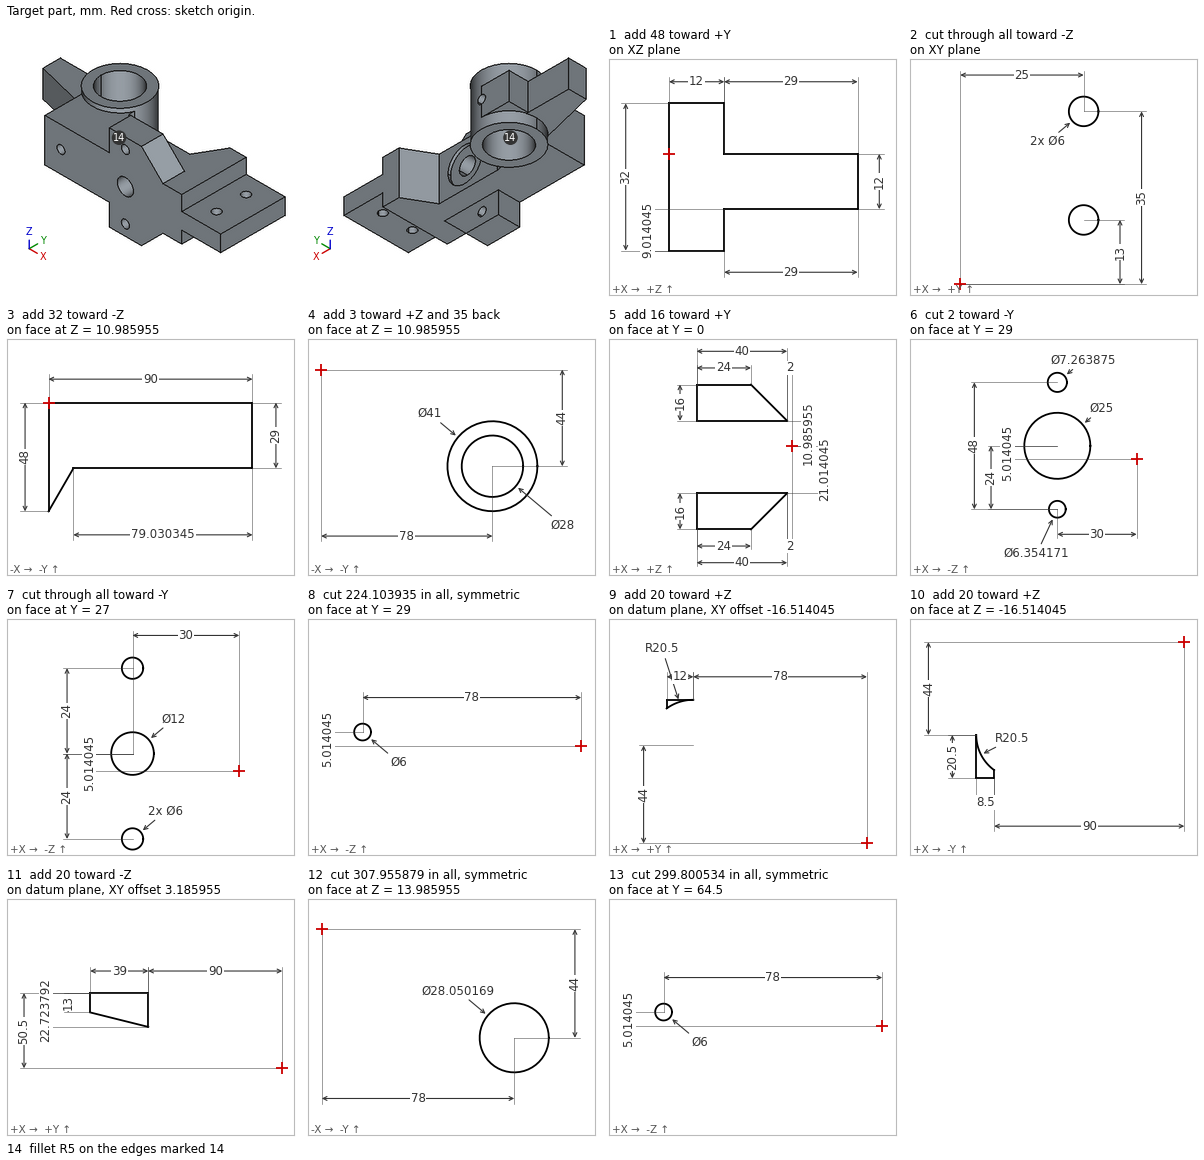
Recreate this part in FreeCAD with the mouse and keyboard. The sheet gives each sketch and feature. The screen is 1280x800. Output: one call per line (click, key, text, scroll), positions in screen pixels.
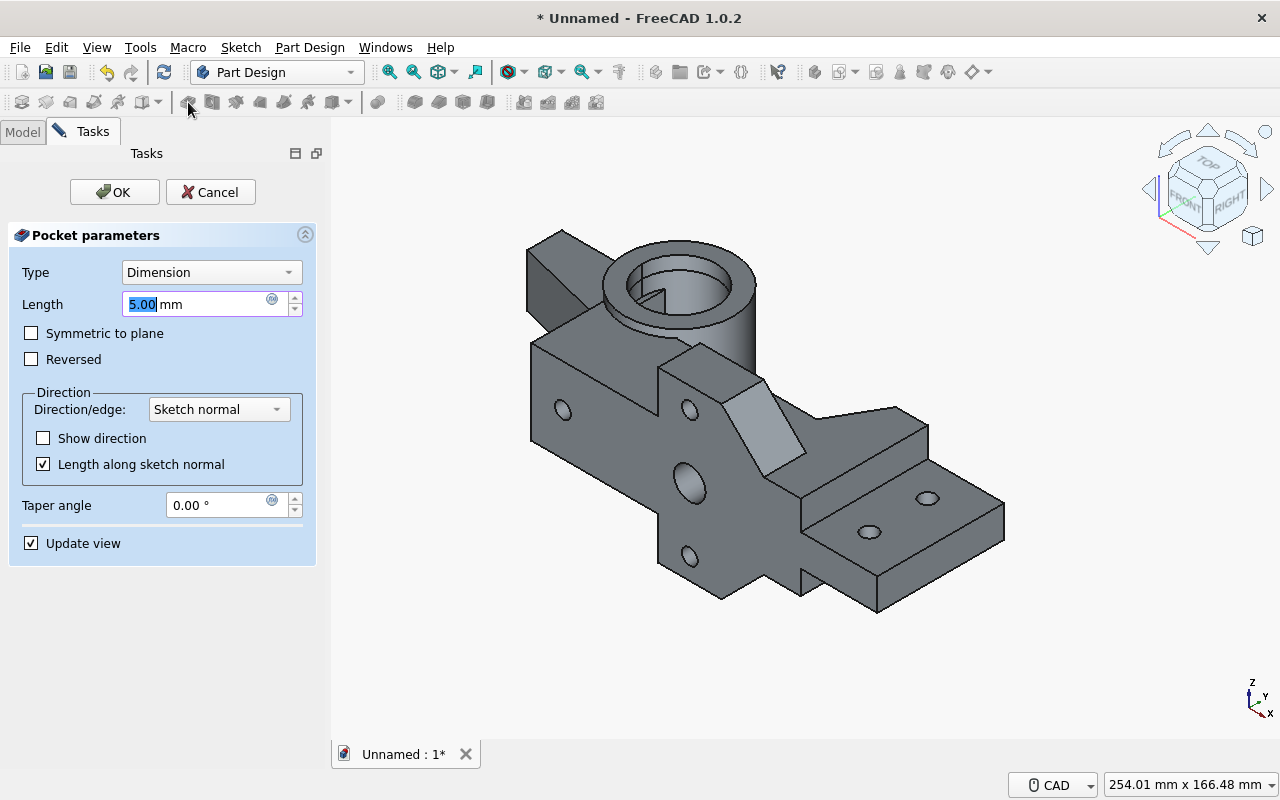
text(307.955879)
key(Tab)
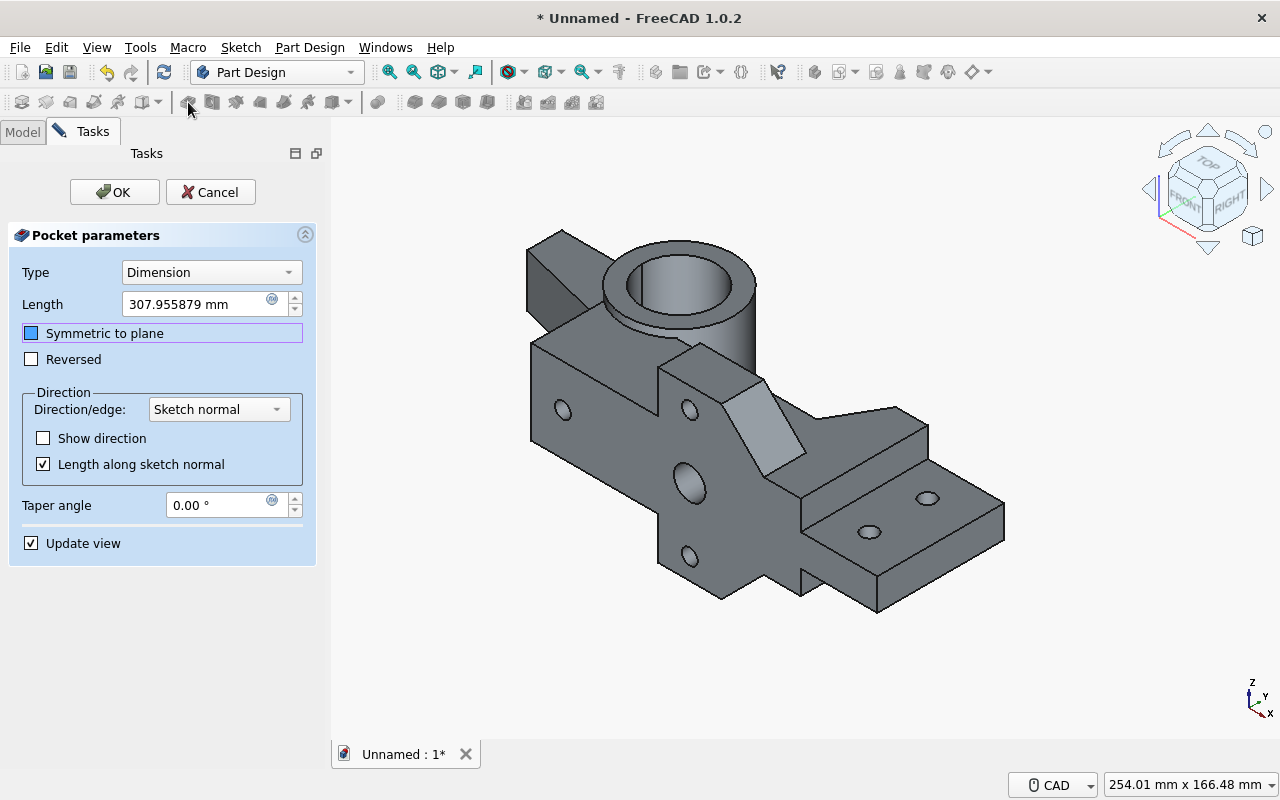
click(30, 333)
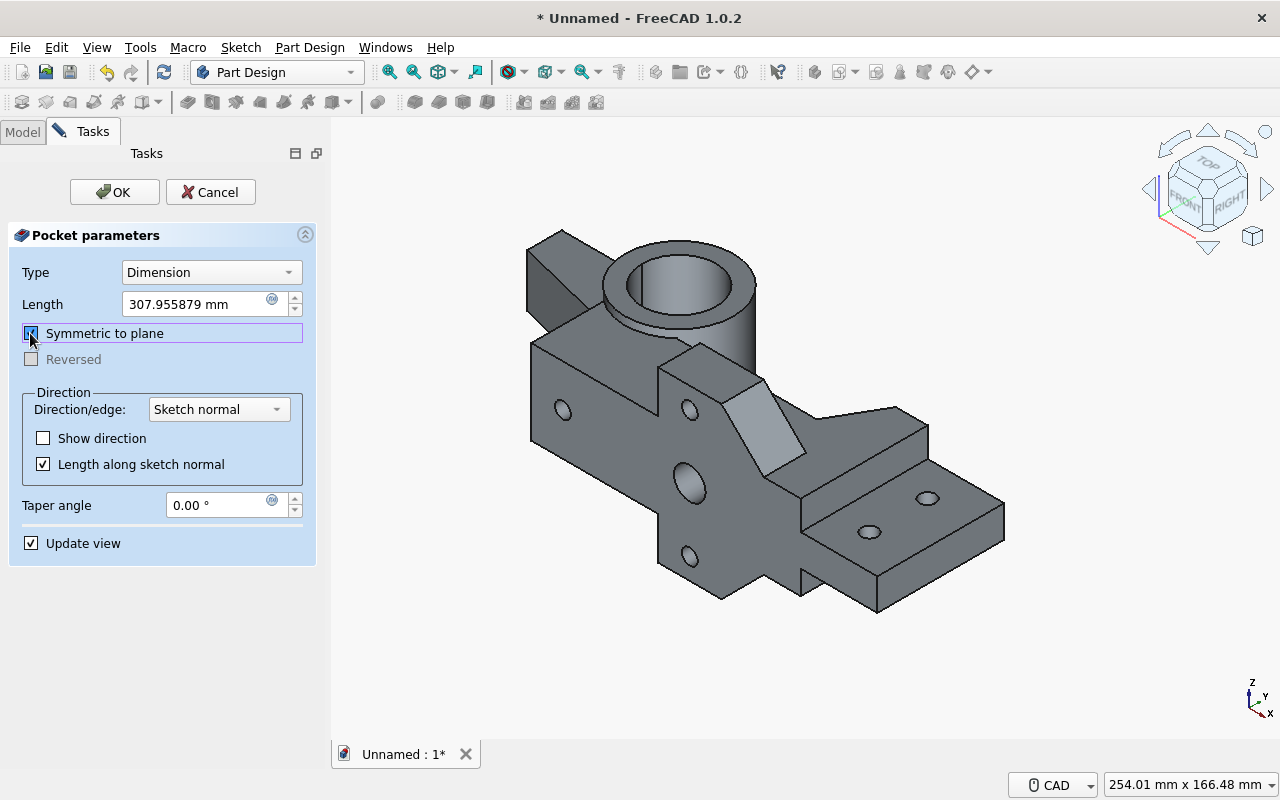
click(115, 192)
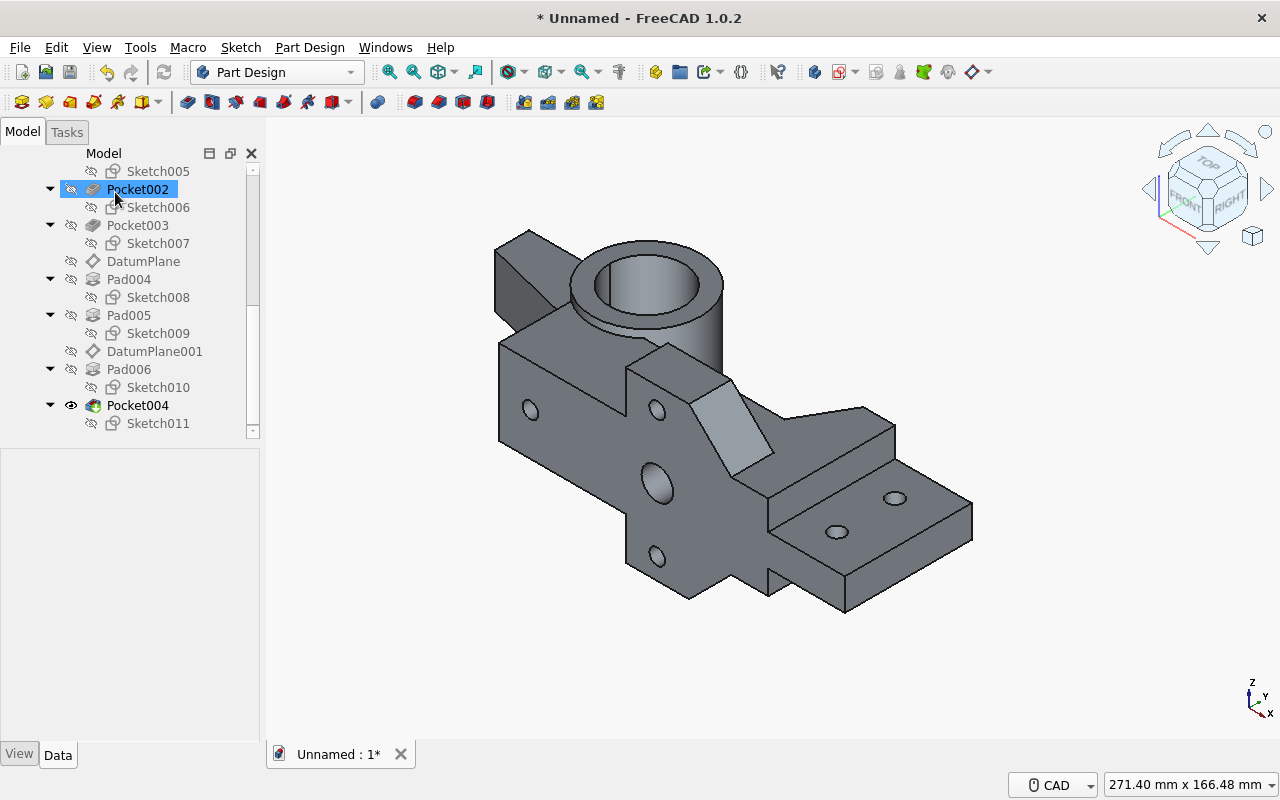
key(4)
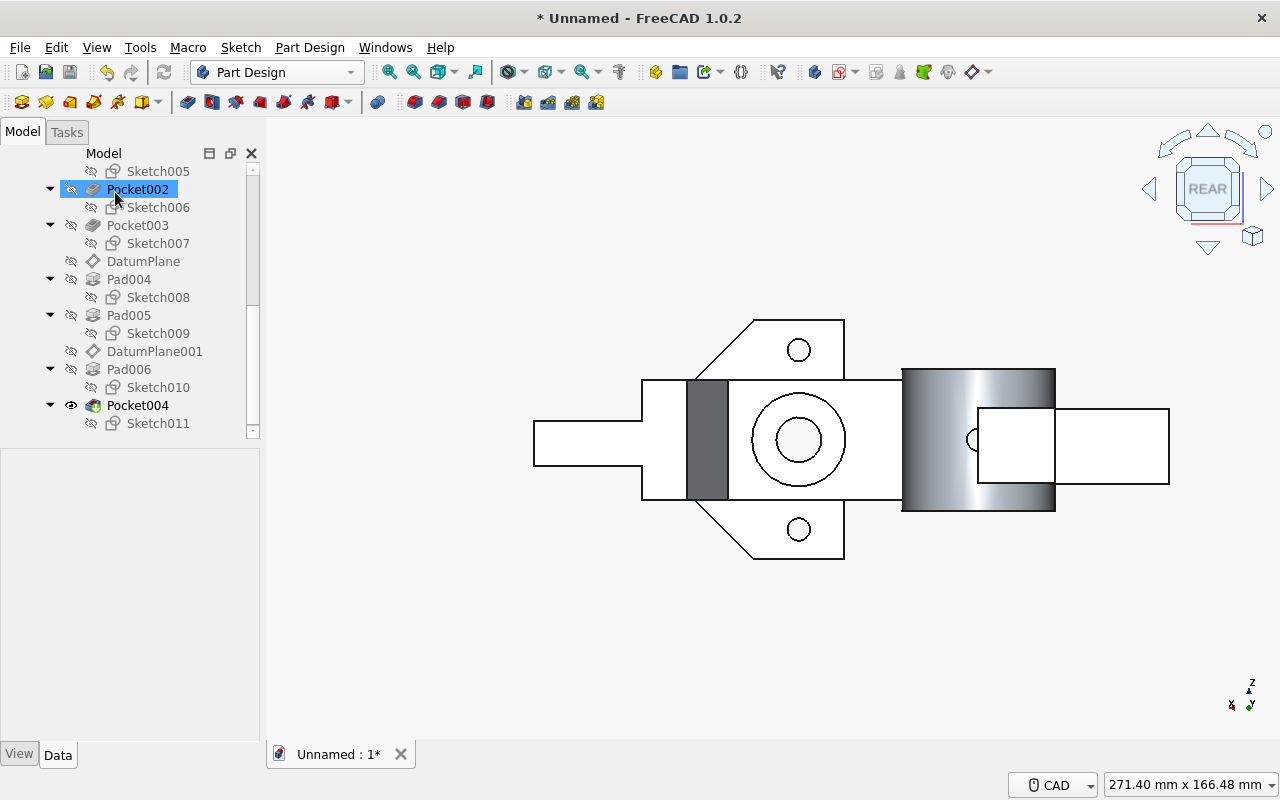
click(1016, 444)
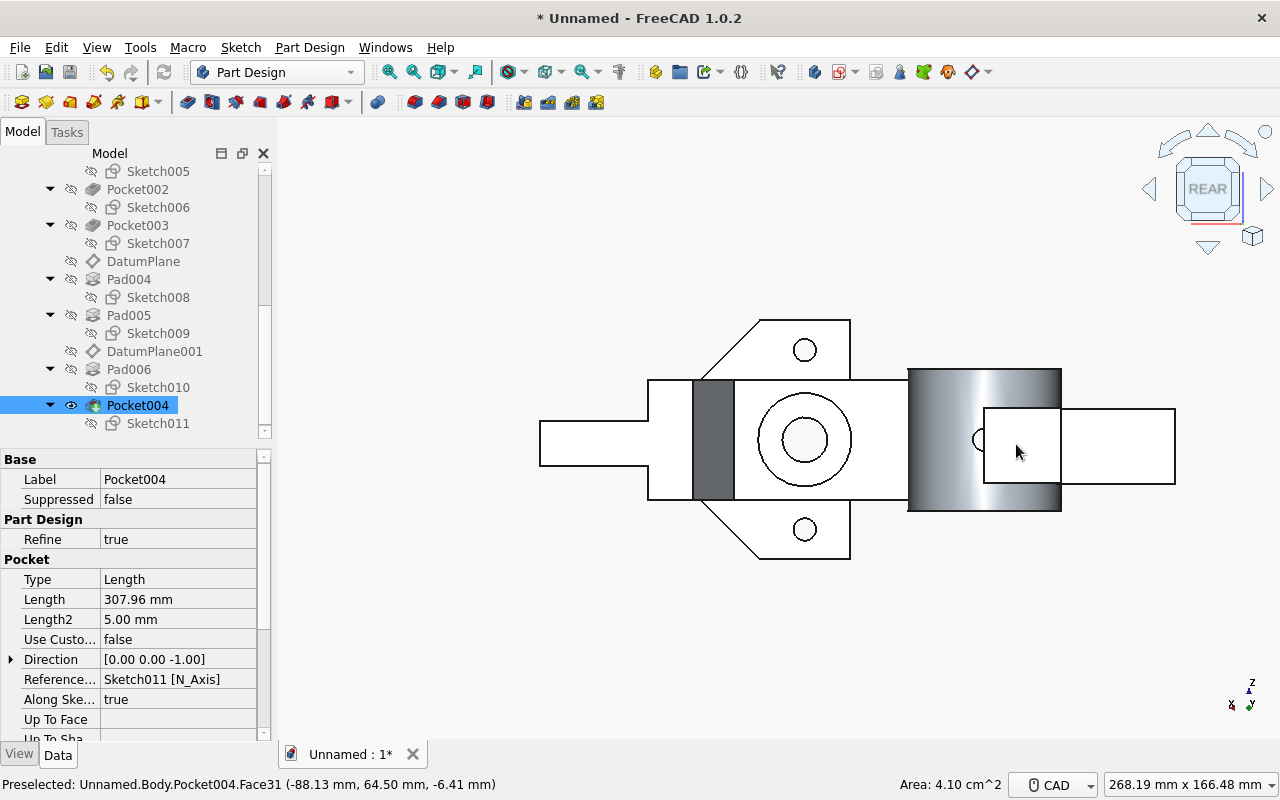
click(840, 72)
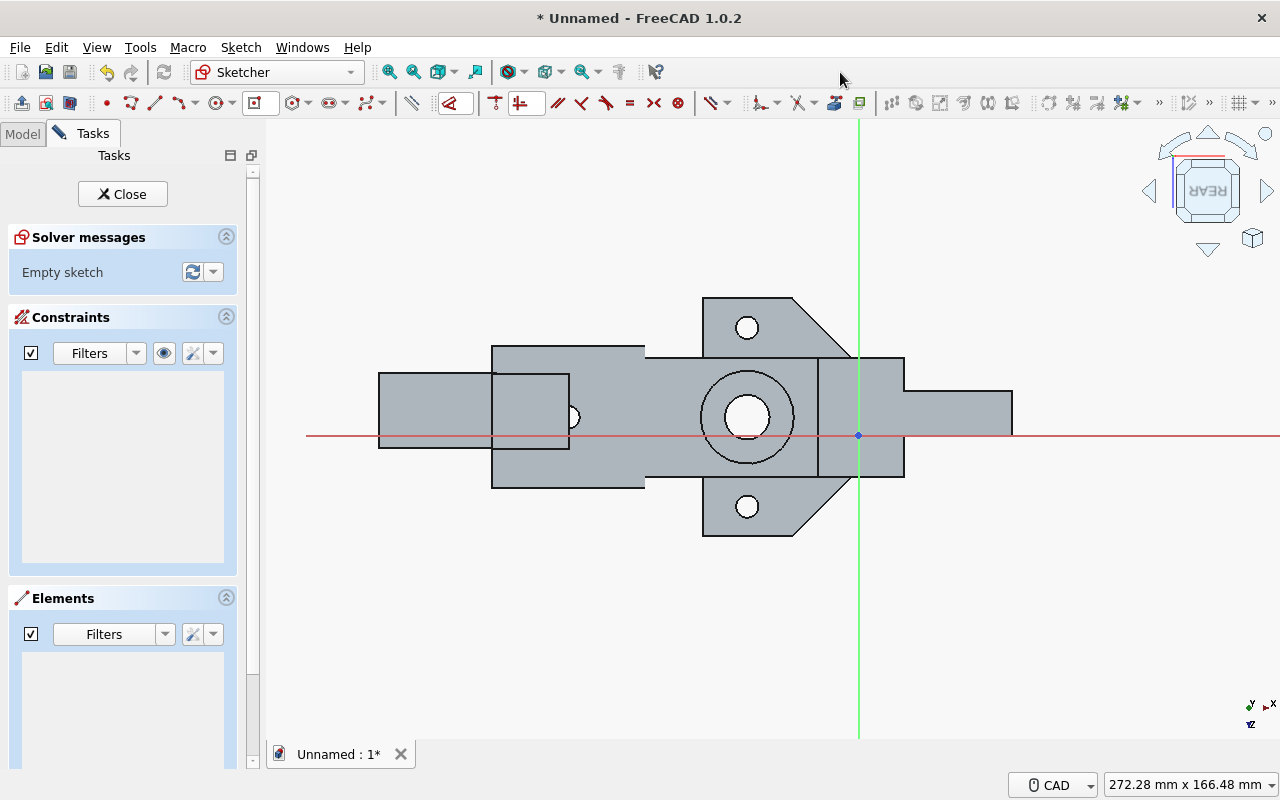
scroll(560, 416, up, 14)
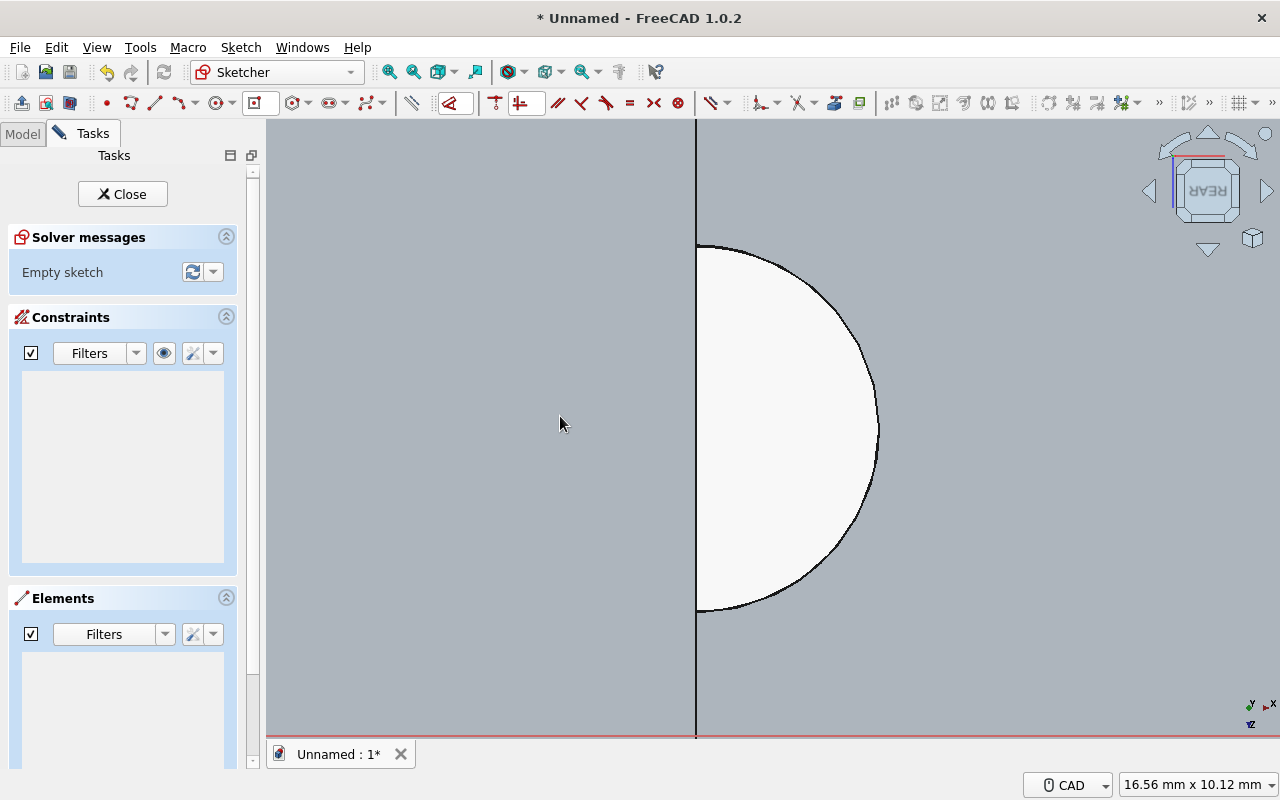
key(g)
key(c)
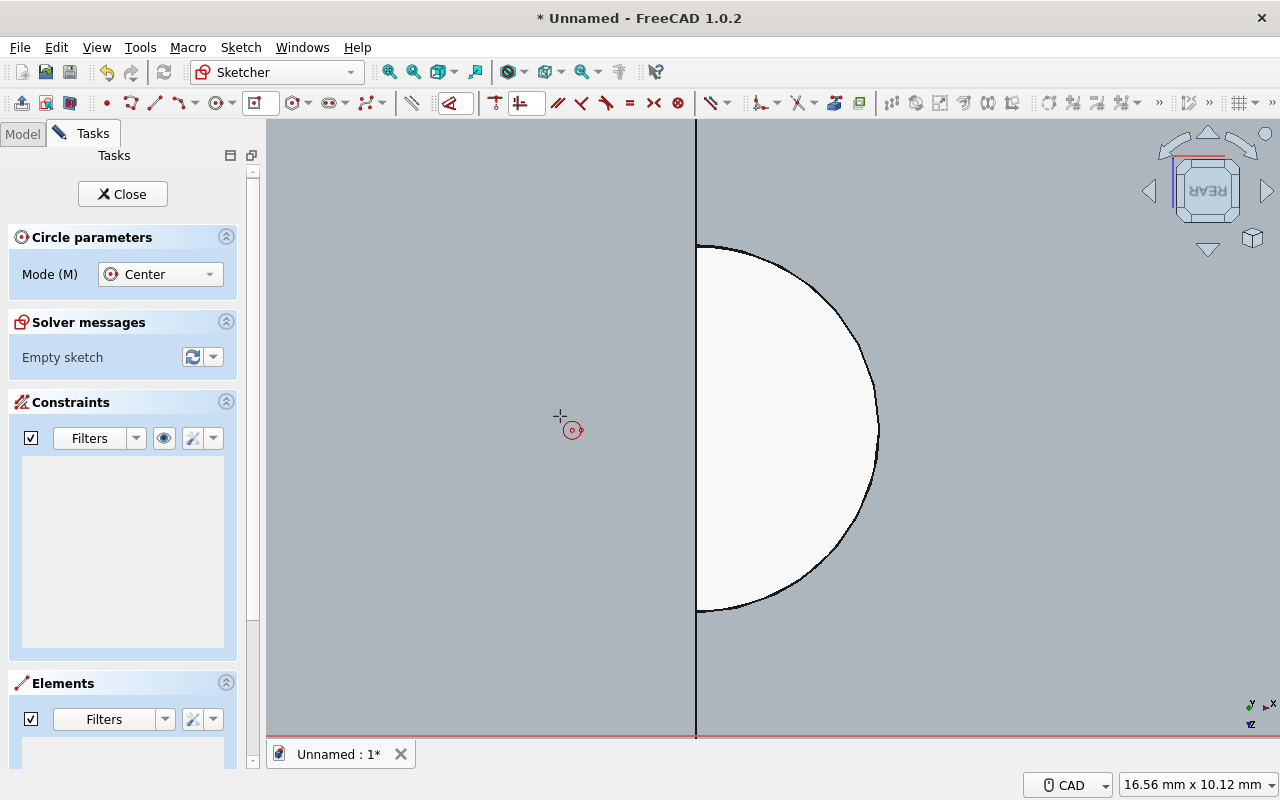
click(696, 429)
move(825, 299)